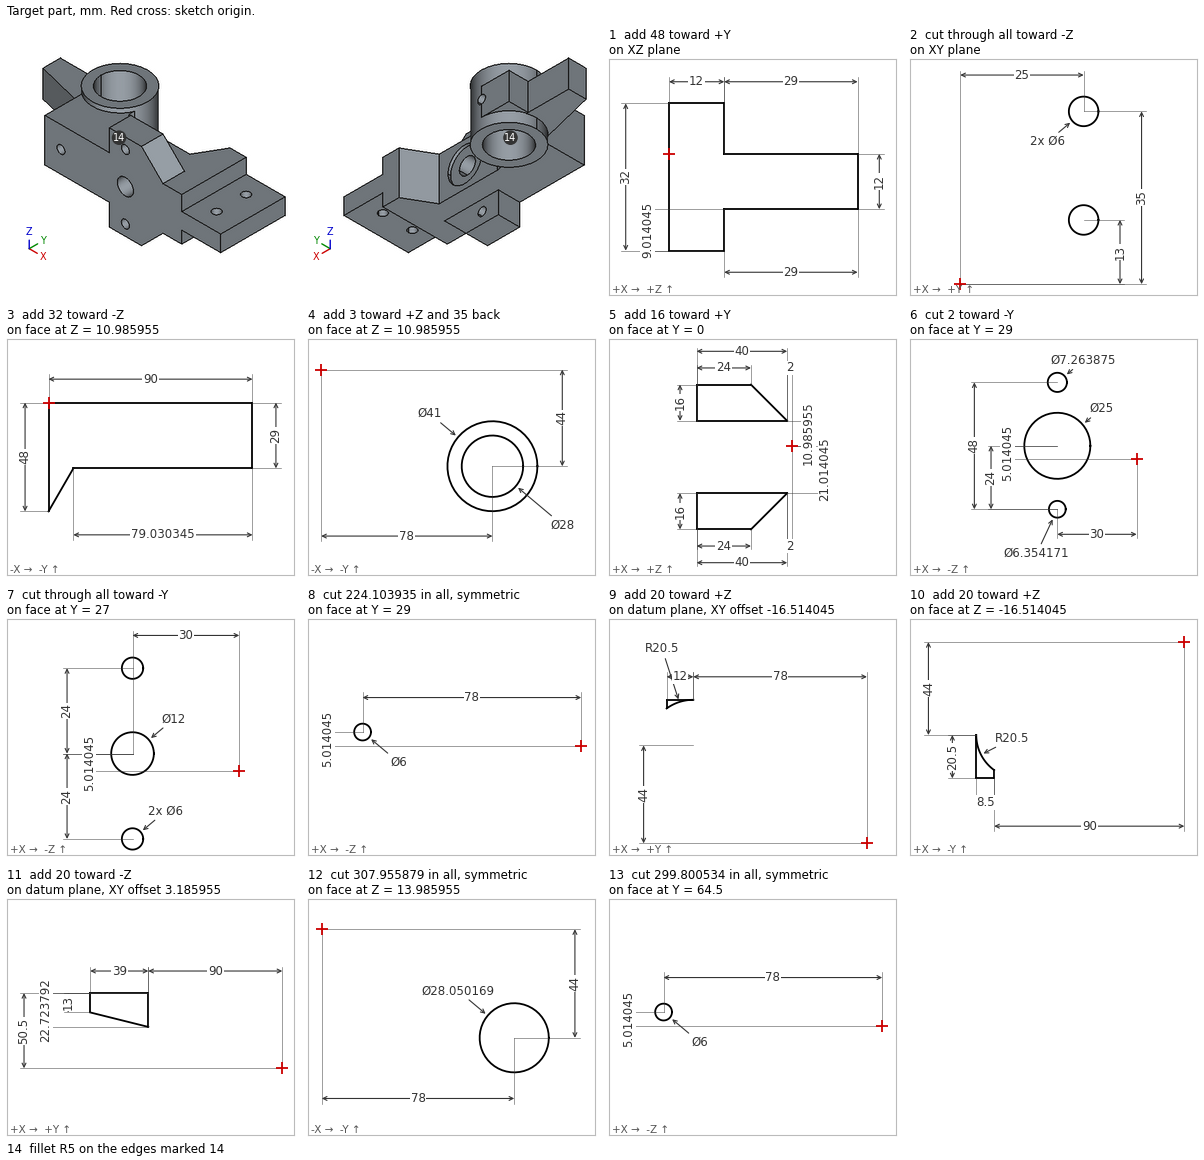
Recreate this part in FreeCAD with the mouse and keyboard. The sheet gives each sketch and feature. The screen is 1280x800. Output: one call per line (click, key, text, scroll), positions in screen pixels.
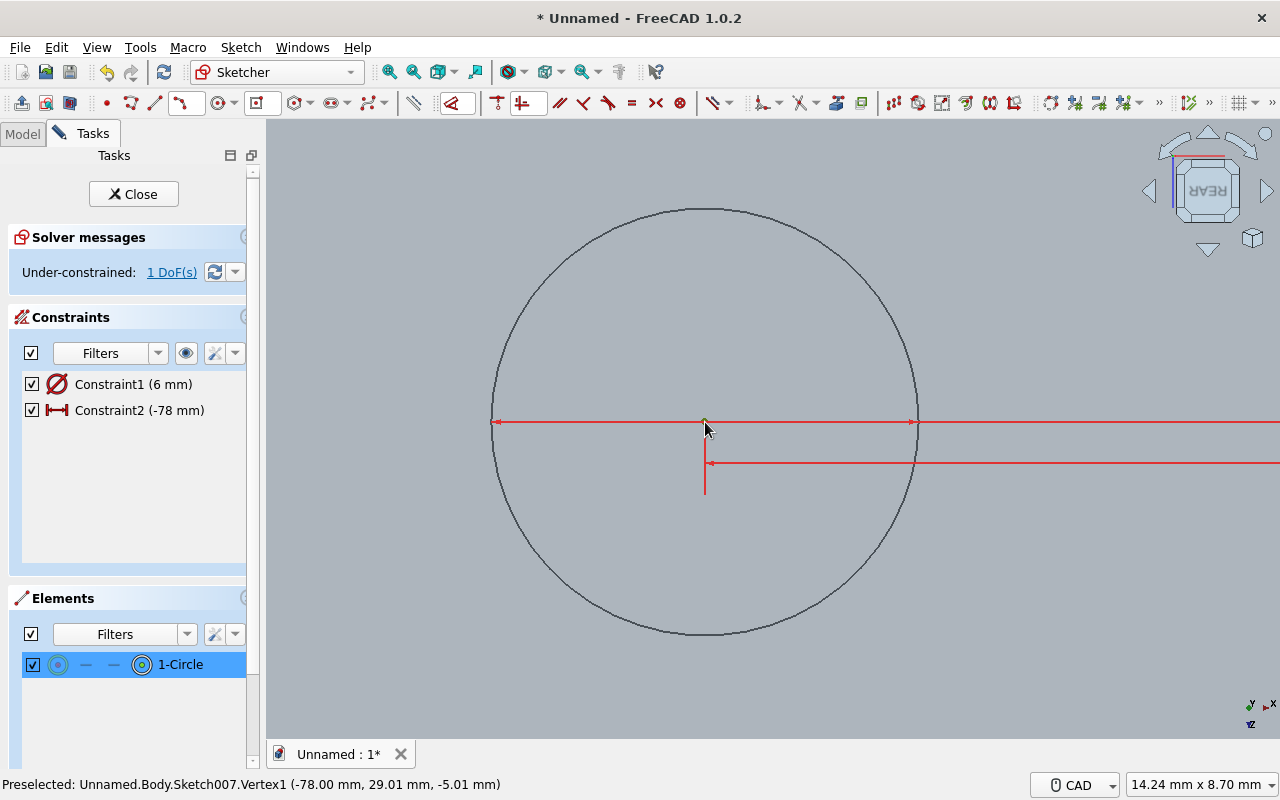
key(i)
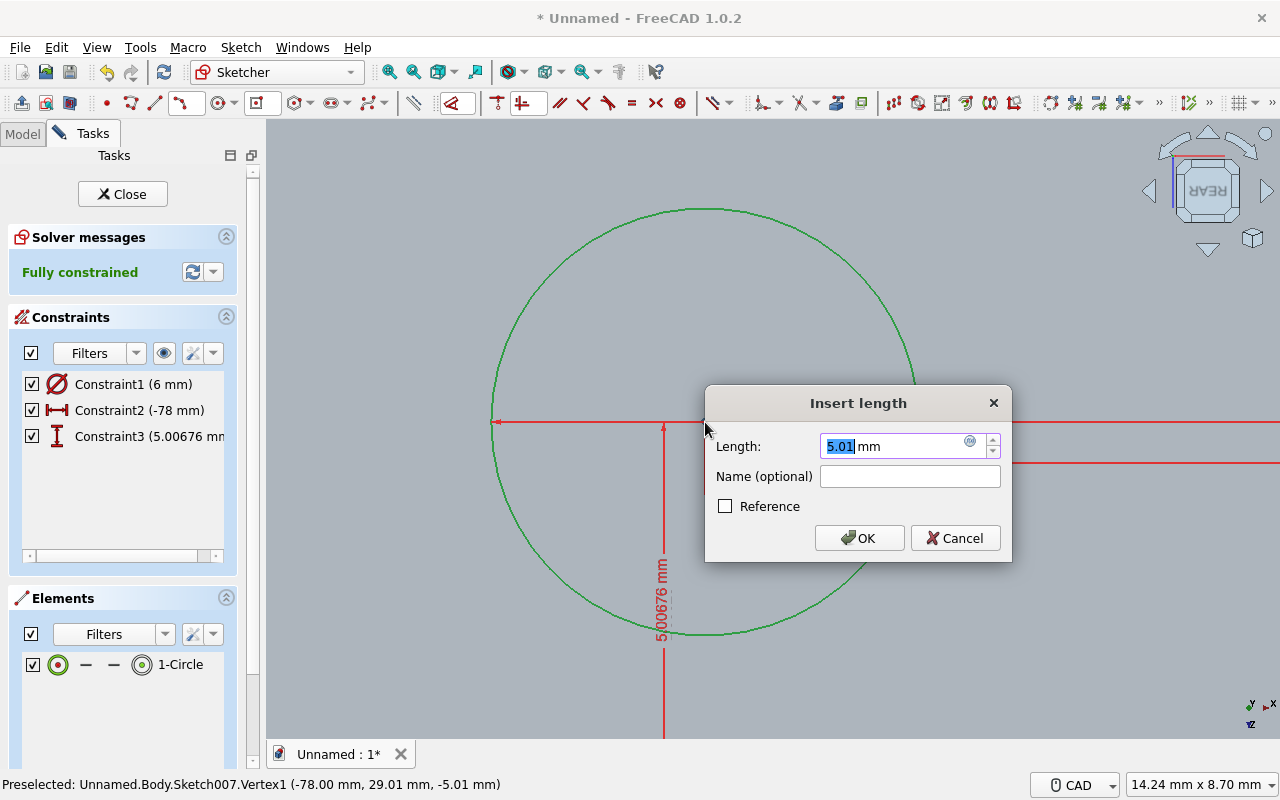
text(5.014045)
key(Return)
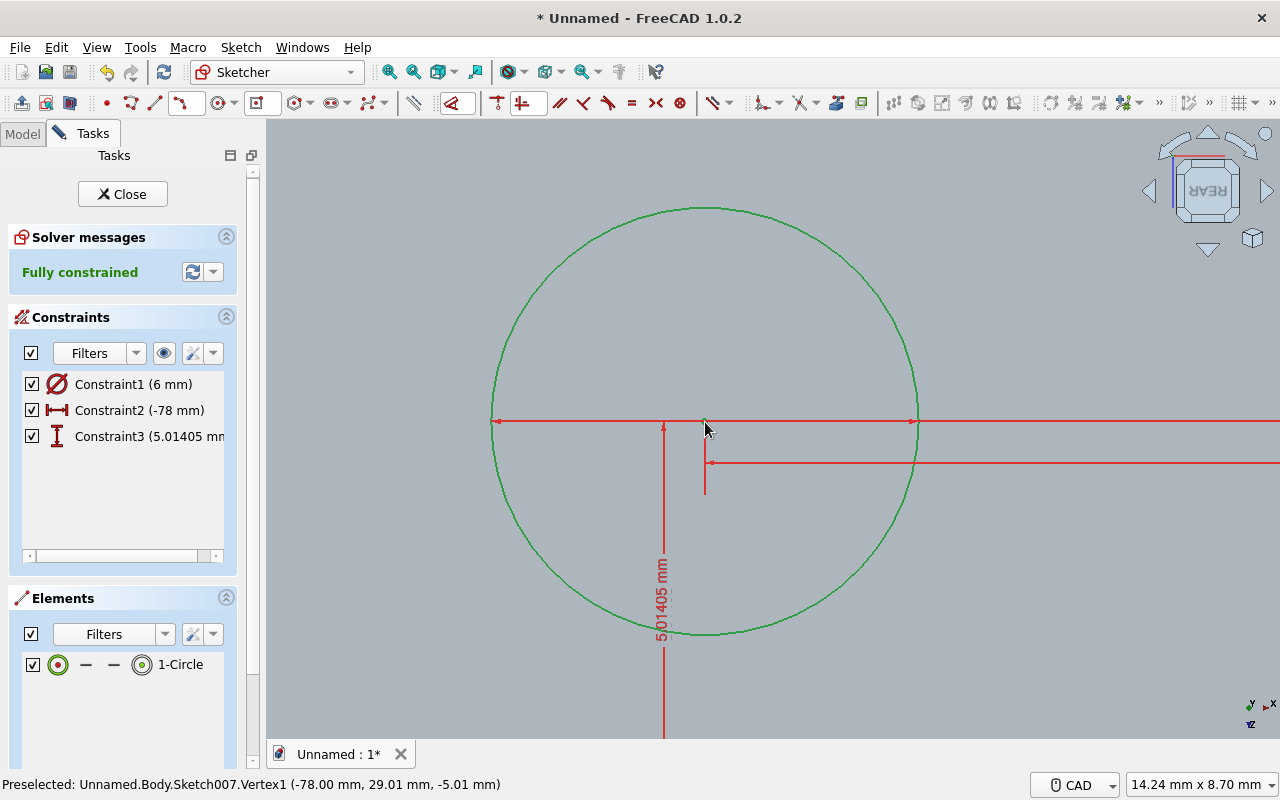
click(123, 194)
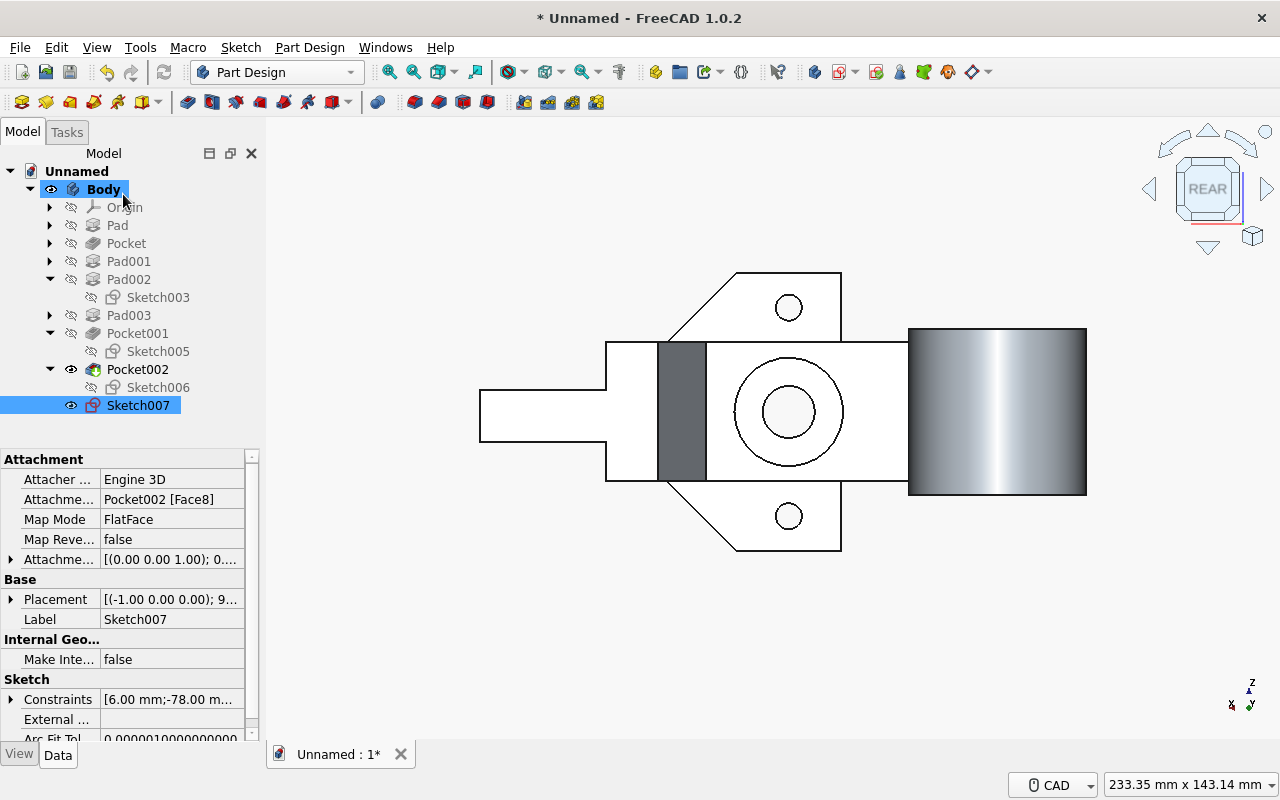
click(188, 102)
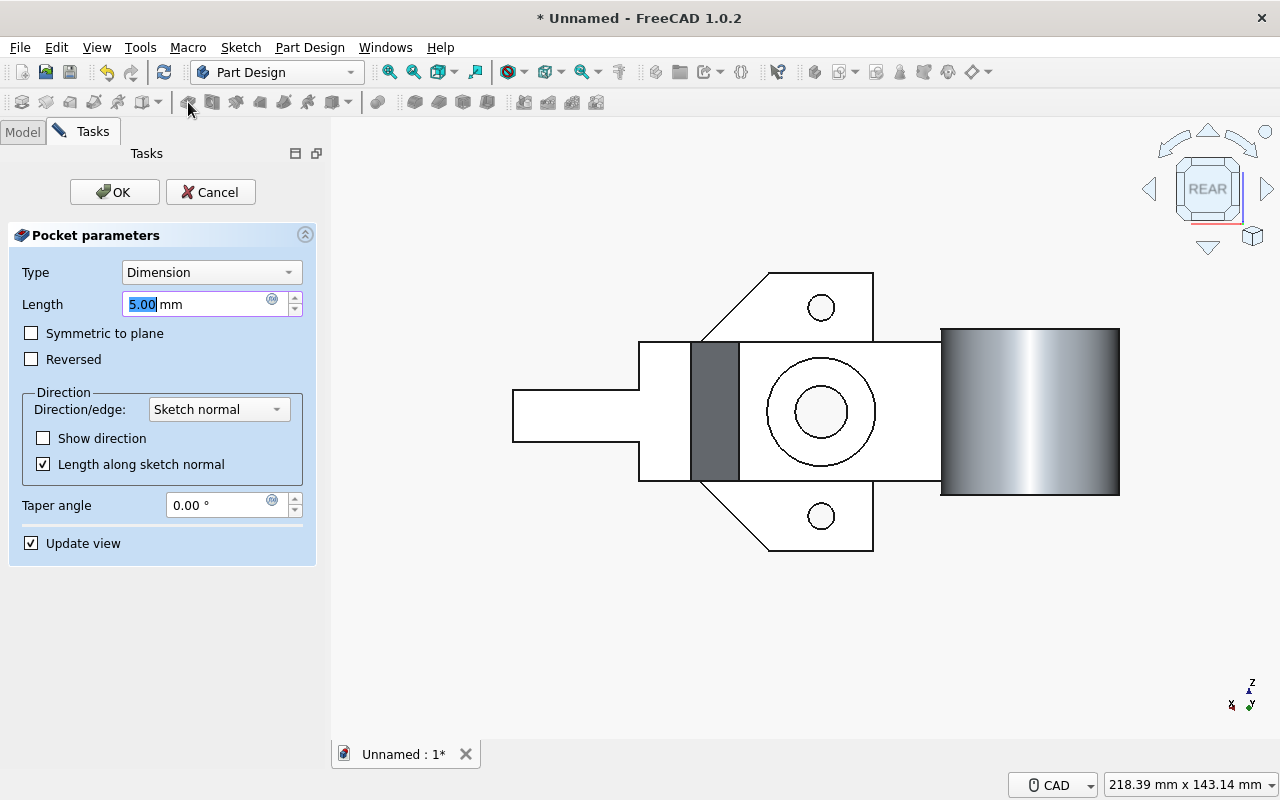
text(224.103935)
key(Tab)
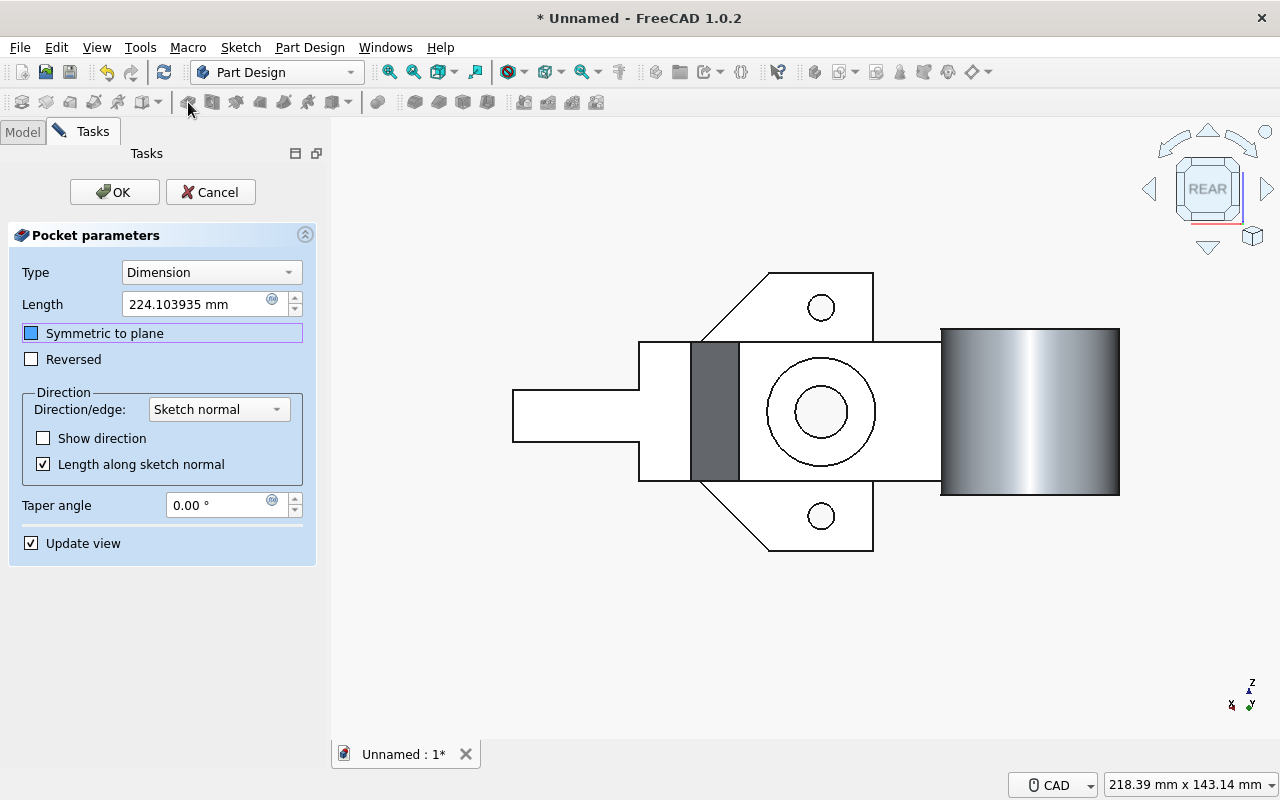
click(30, 333)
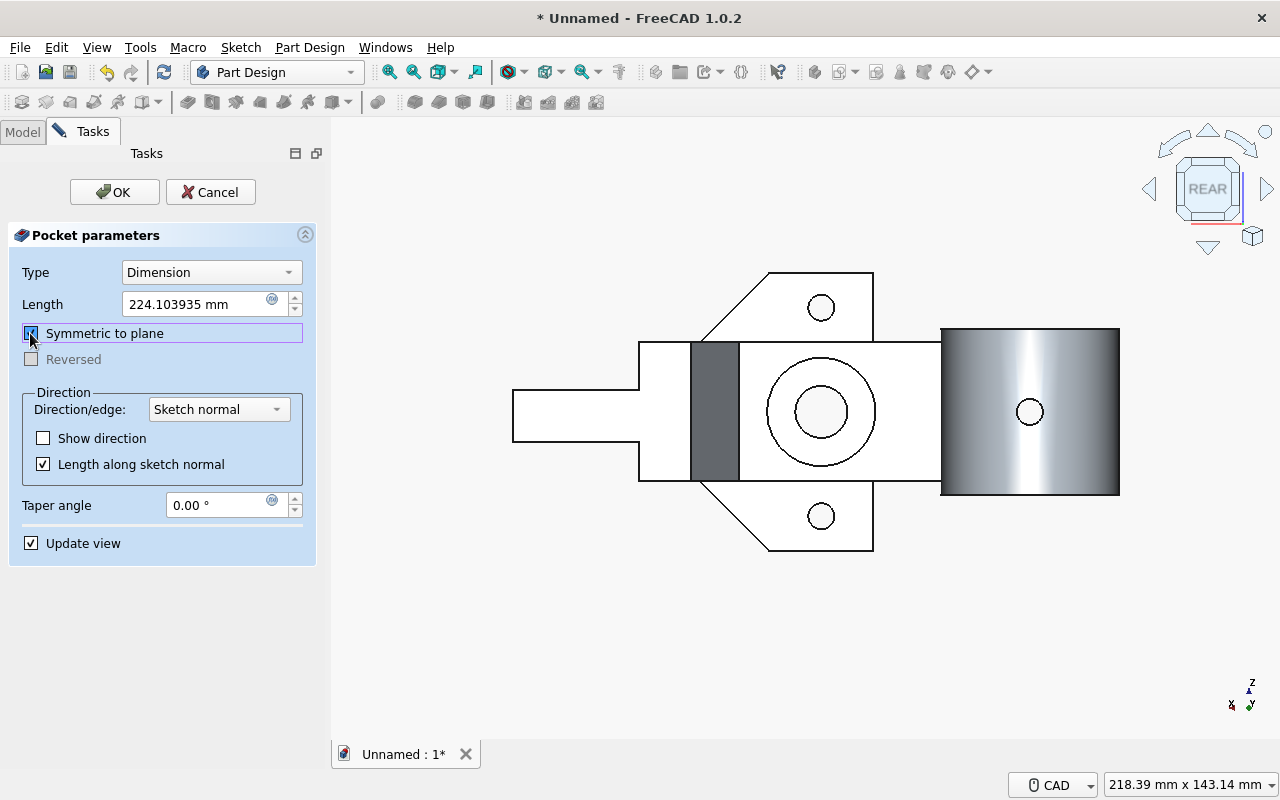
click(115, 192)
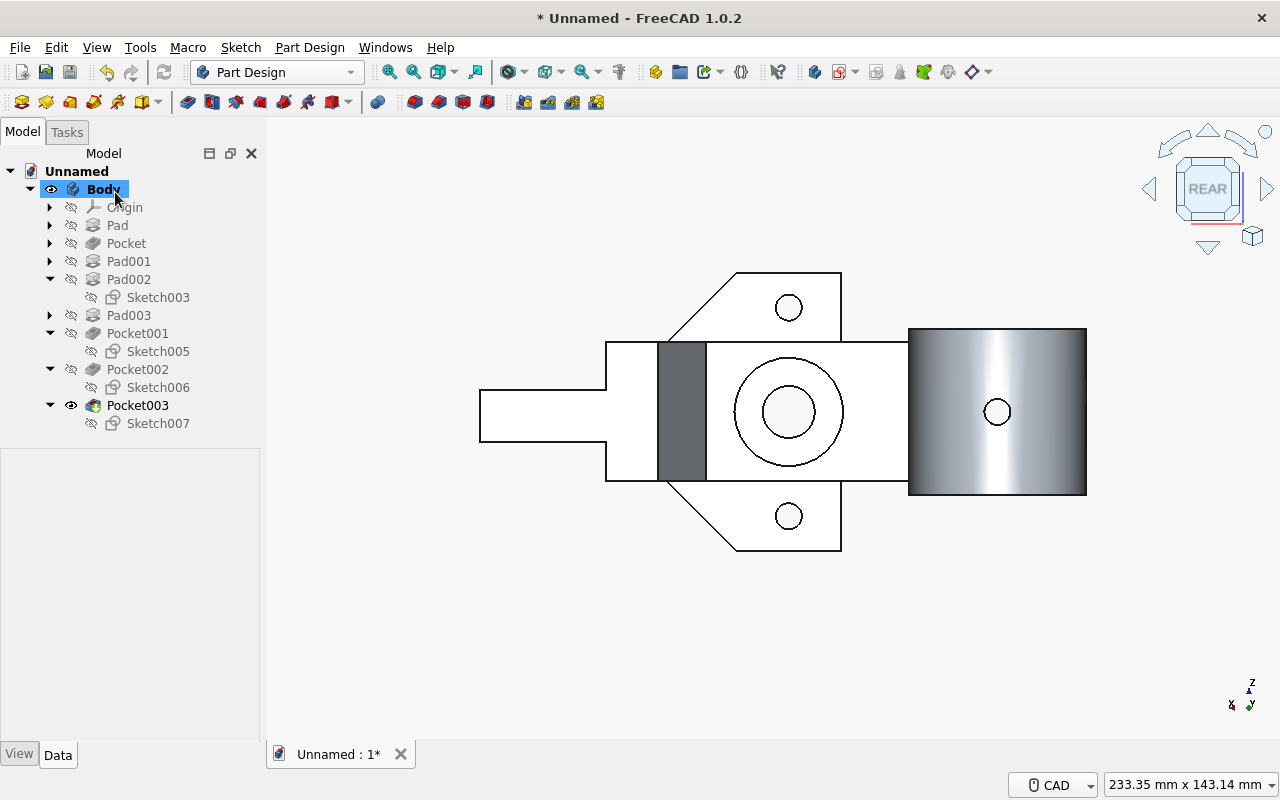
click(50, 207)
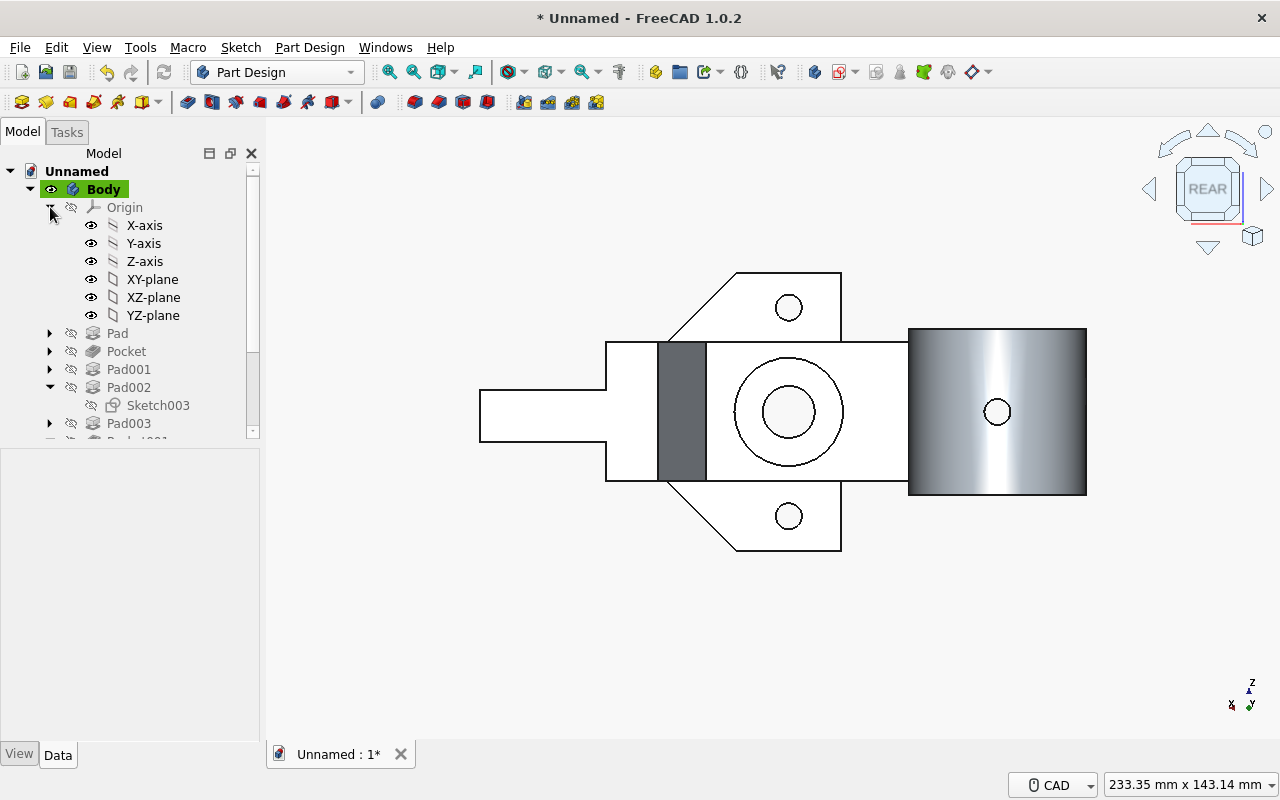
click(136, 279)